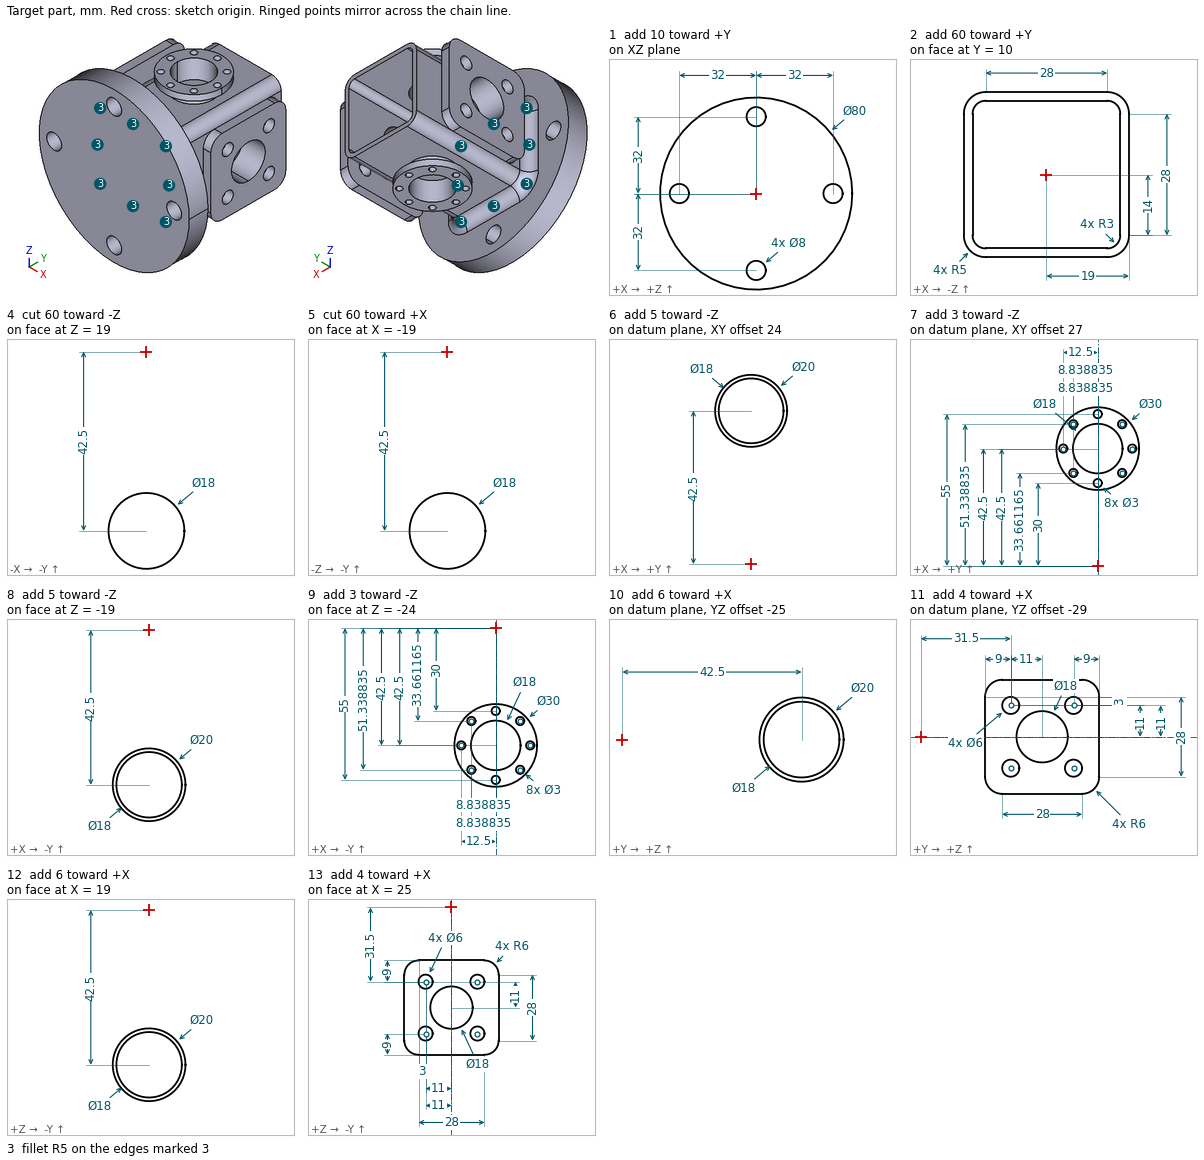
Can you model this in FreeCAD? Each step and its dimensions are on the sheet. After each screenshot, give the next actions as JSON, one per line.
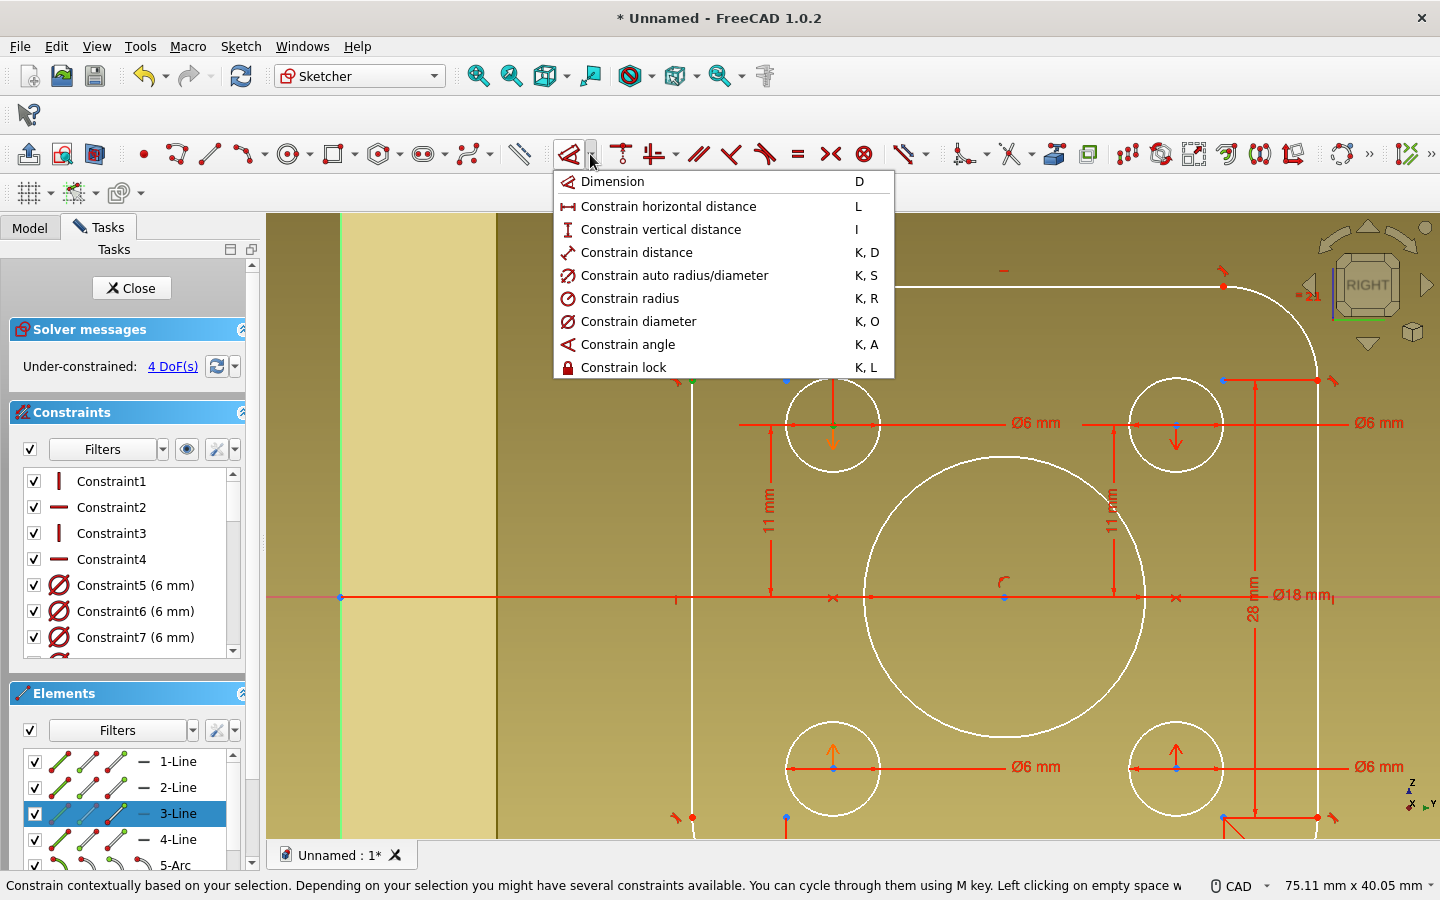
{"action": "left_click", "coordinate": [724, 230]}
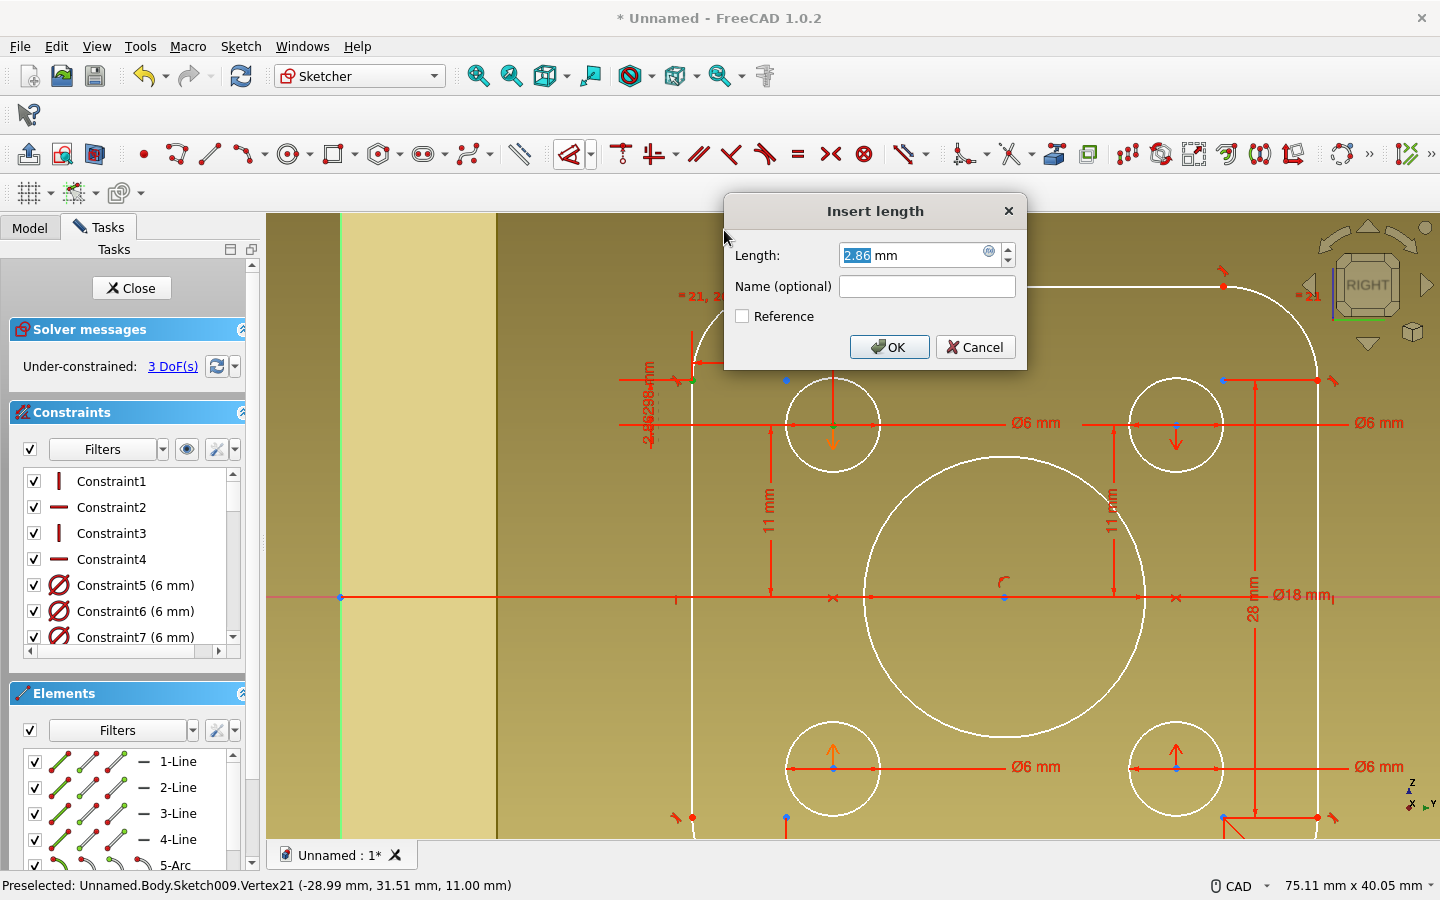
{"action": "type", "text": "3"}
{"action": "key", "text": "Return"}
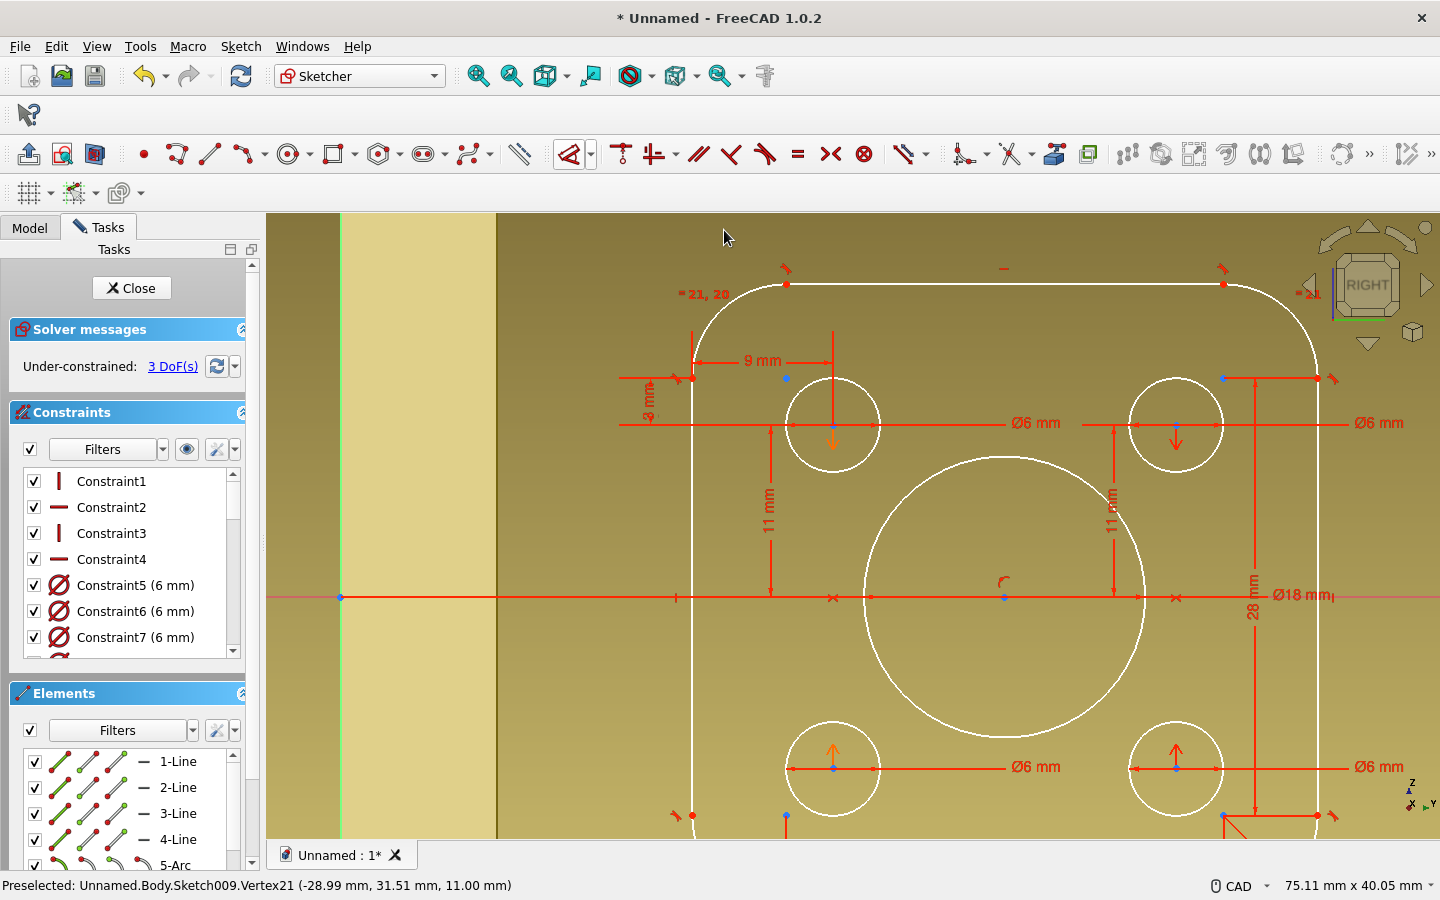
{"action": "scroll", "coordinate": [694, 382], "scroll_direction": "down", "scroll_amount": 2}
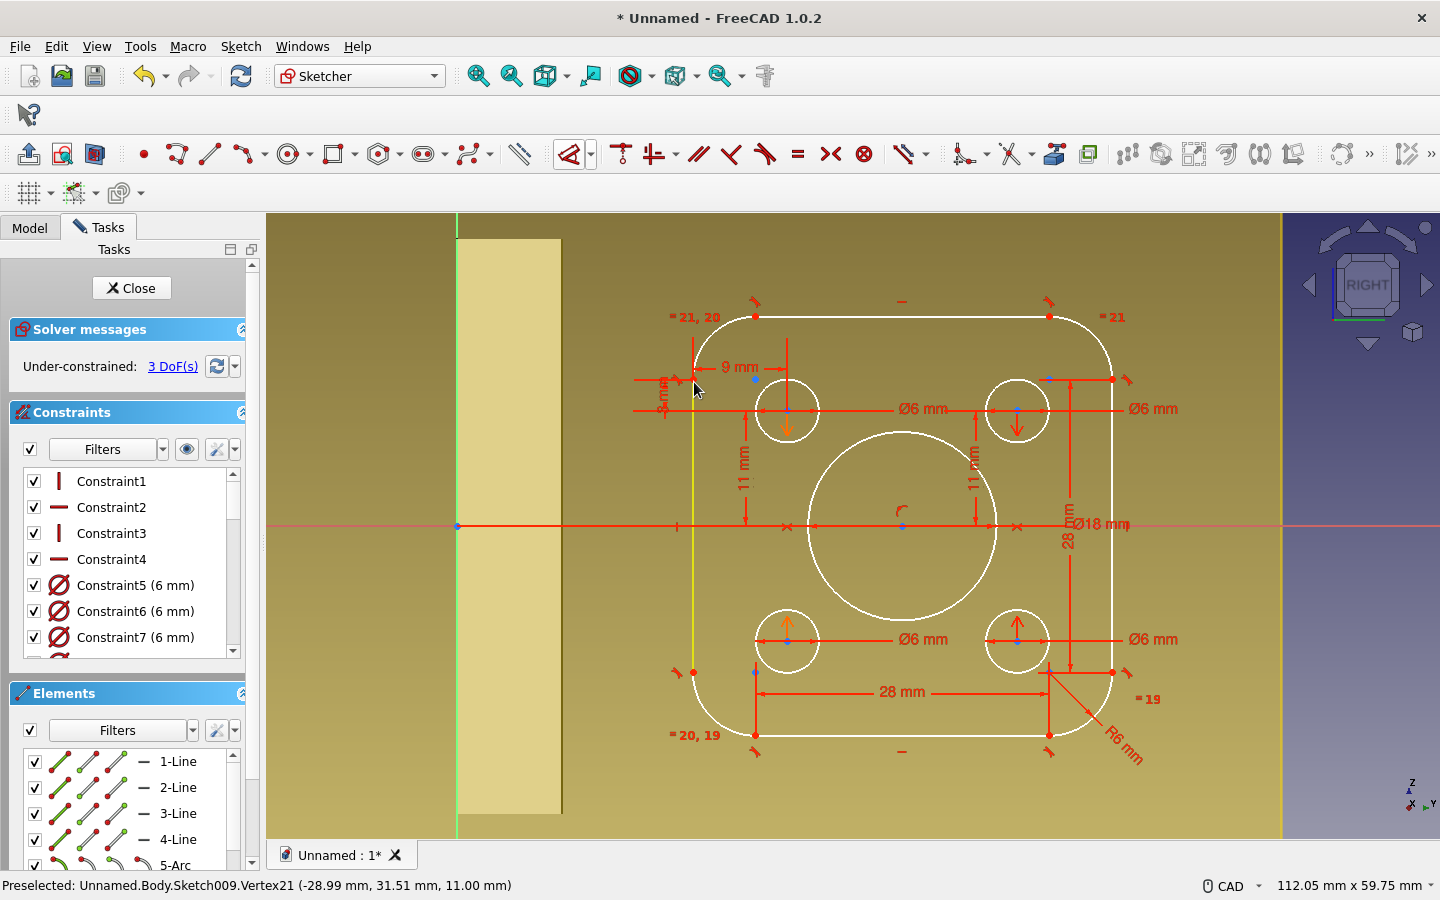
{"action": "left_click", "coordinate": [1112, 380]}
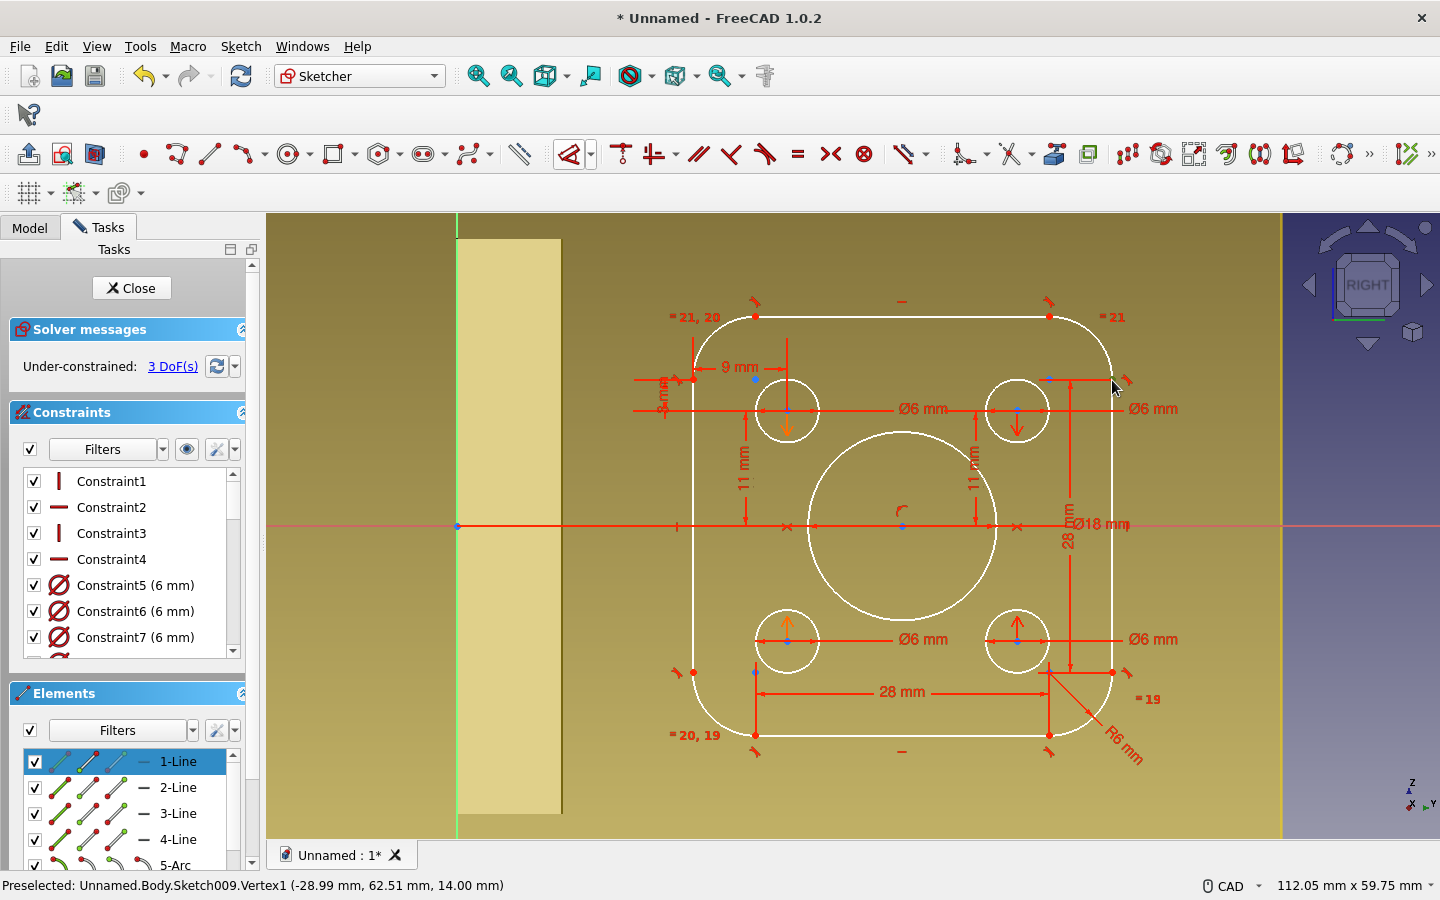
{"action": "left_click", "coordinate": [1017, 411]}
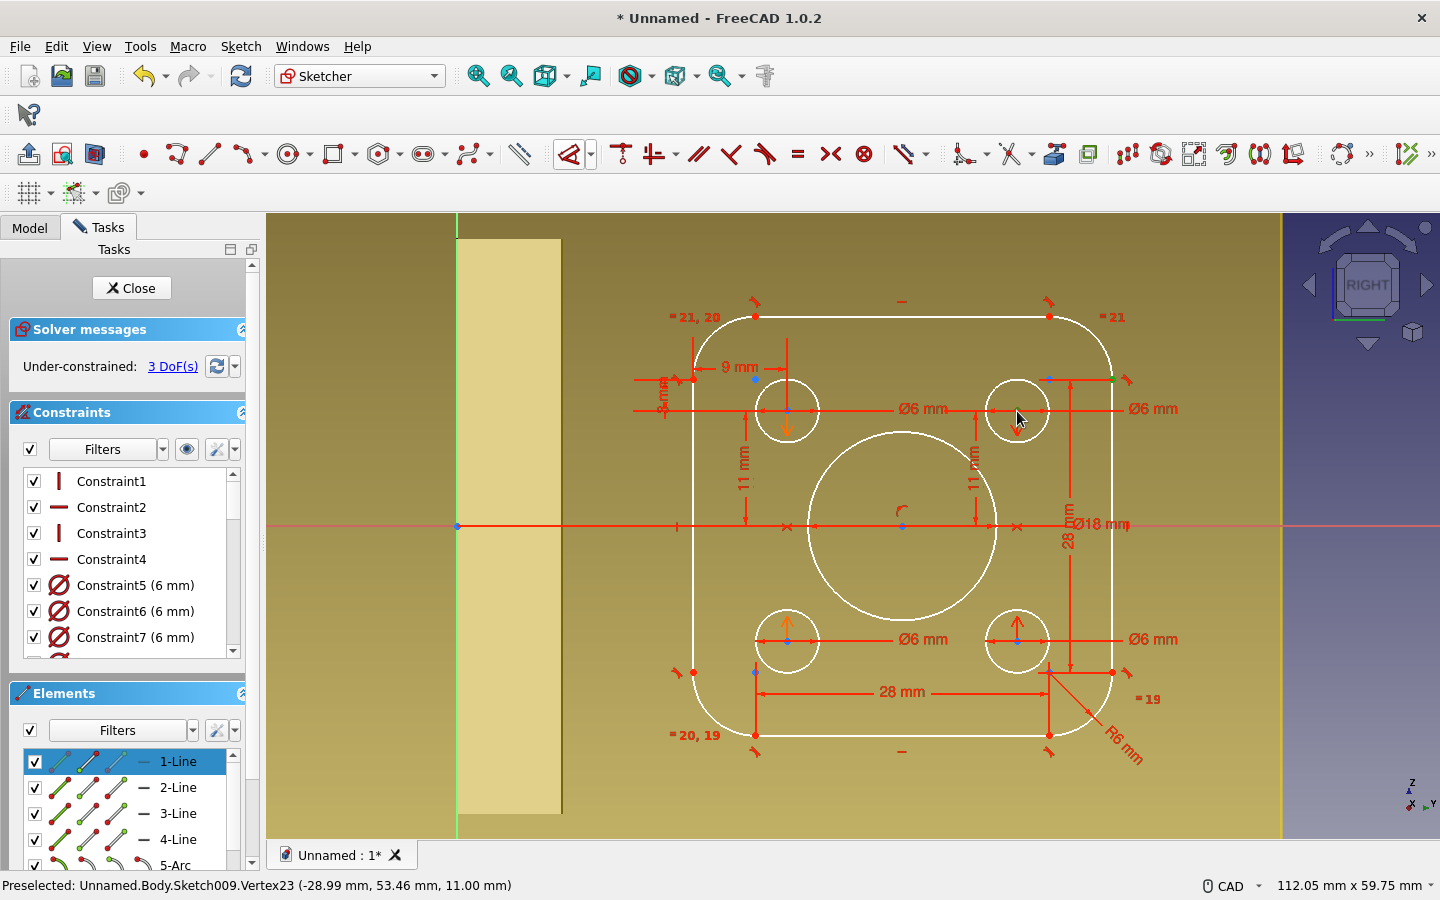
{"action": "key", "text": "l"}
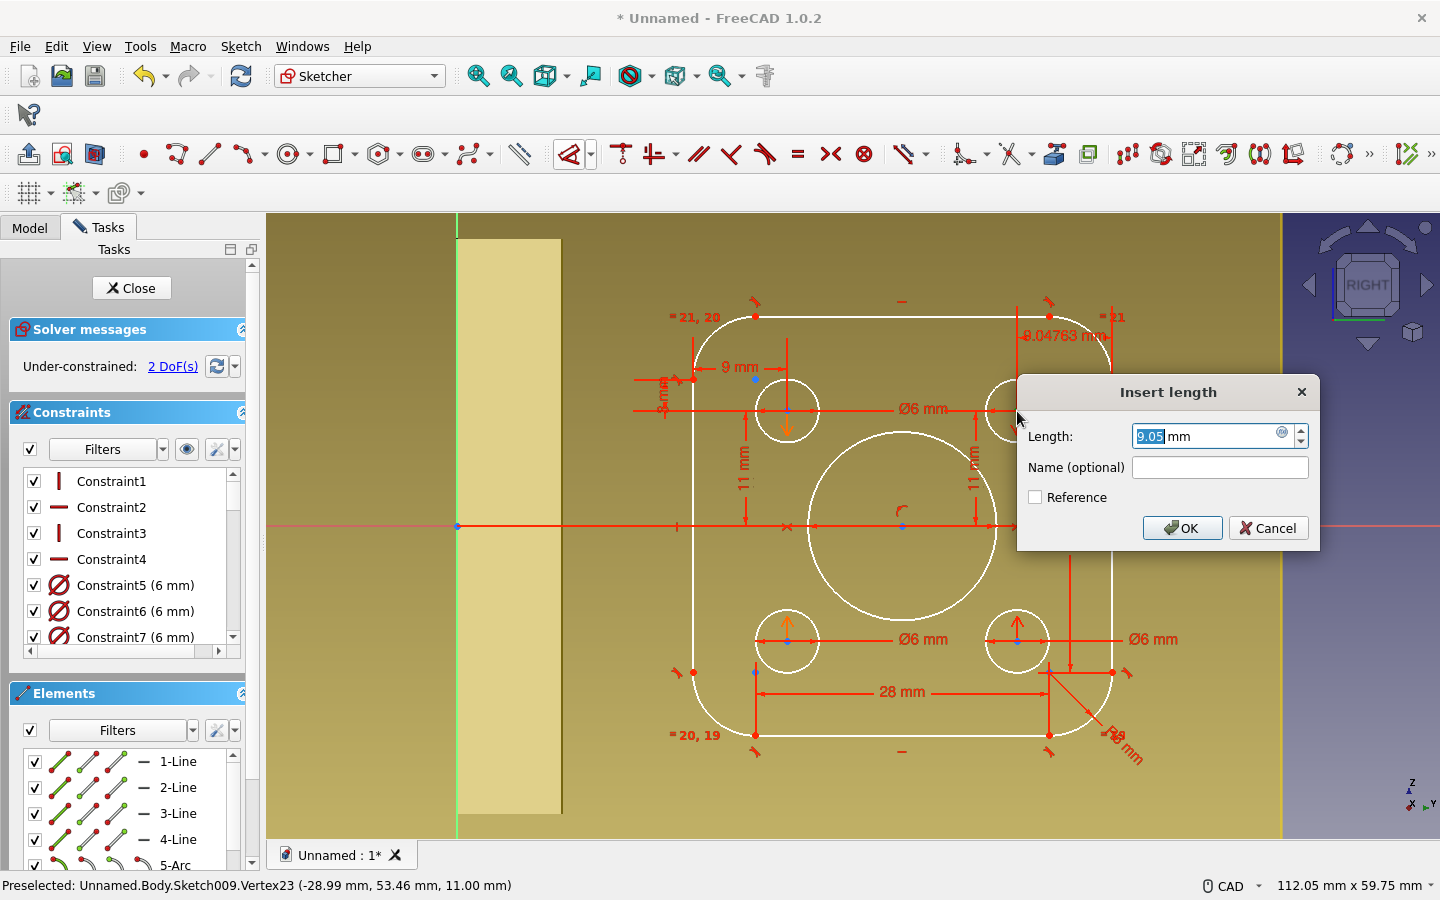
{"action": "type", "text": "9"}
{"action": "key", "text": "Return"}